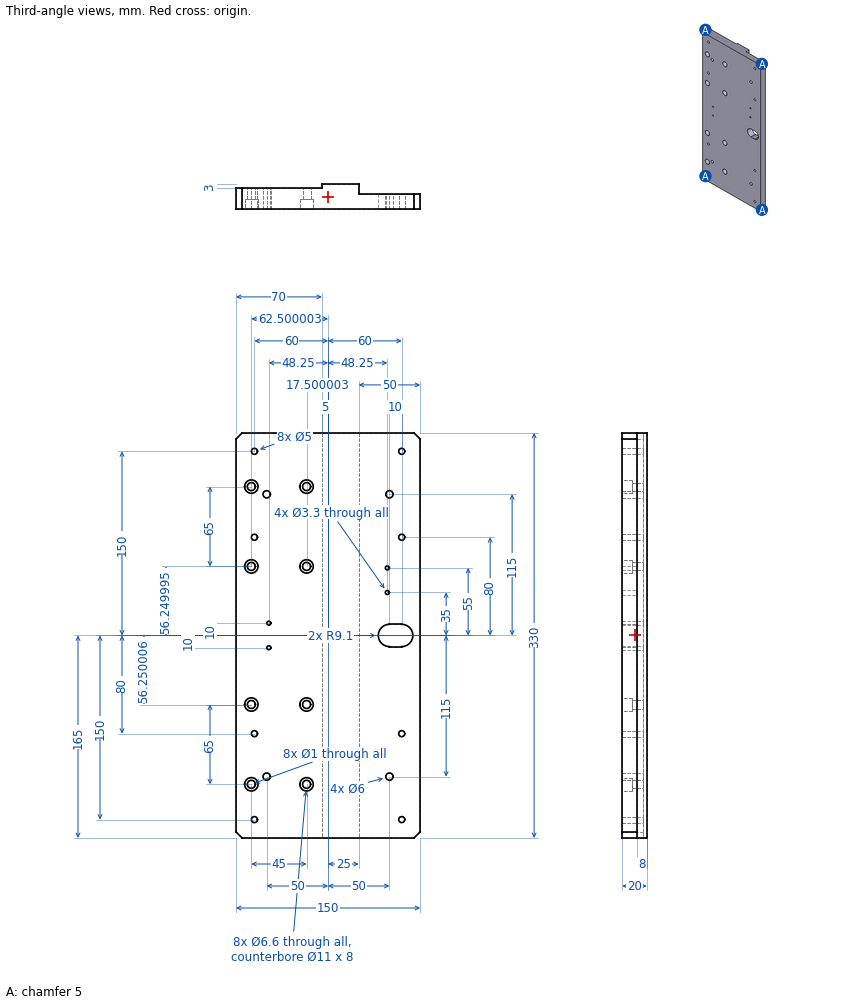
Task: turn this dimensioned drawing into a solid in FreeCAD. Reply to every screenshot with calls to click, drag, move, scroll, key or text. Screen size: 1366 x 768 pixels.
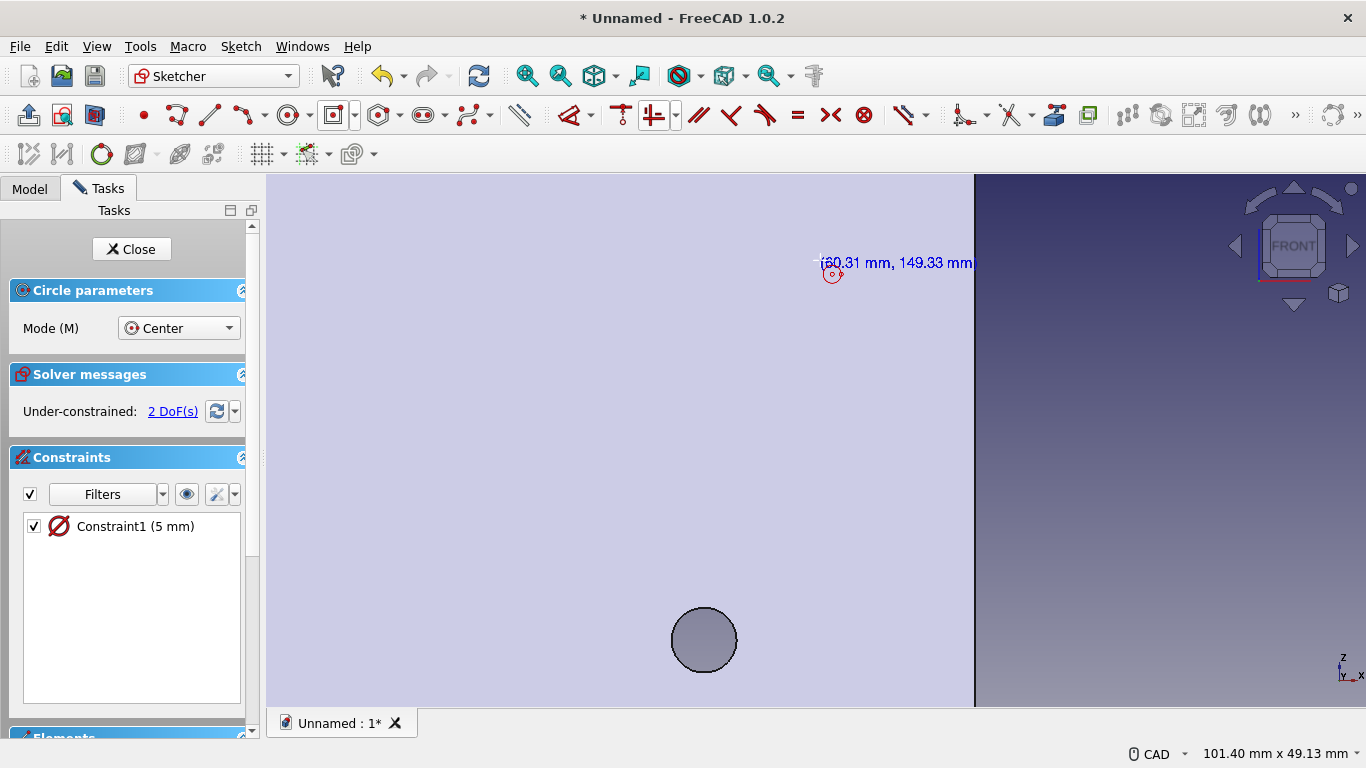
scroll(820, 260, down, 11)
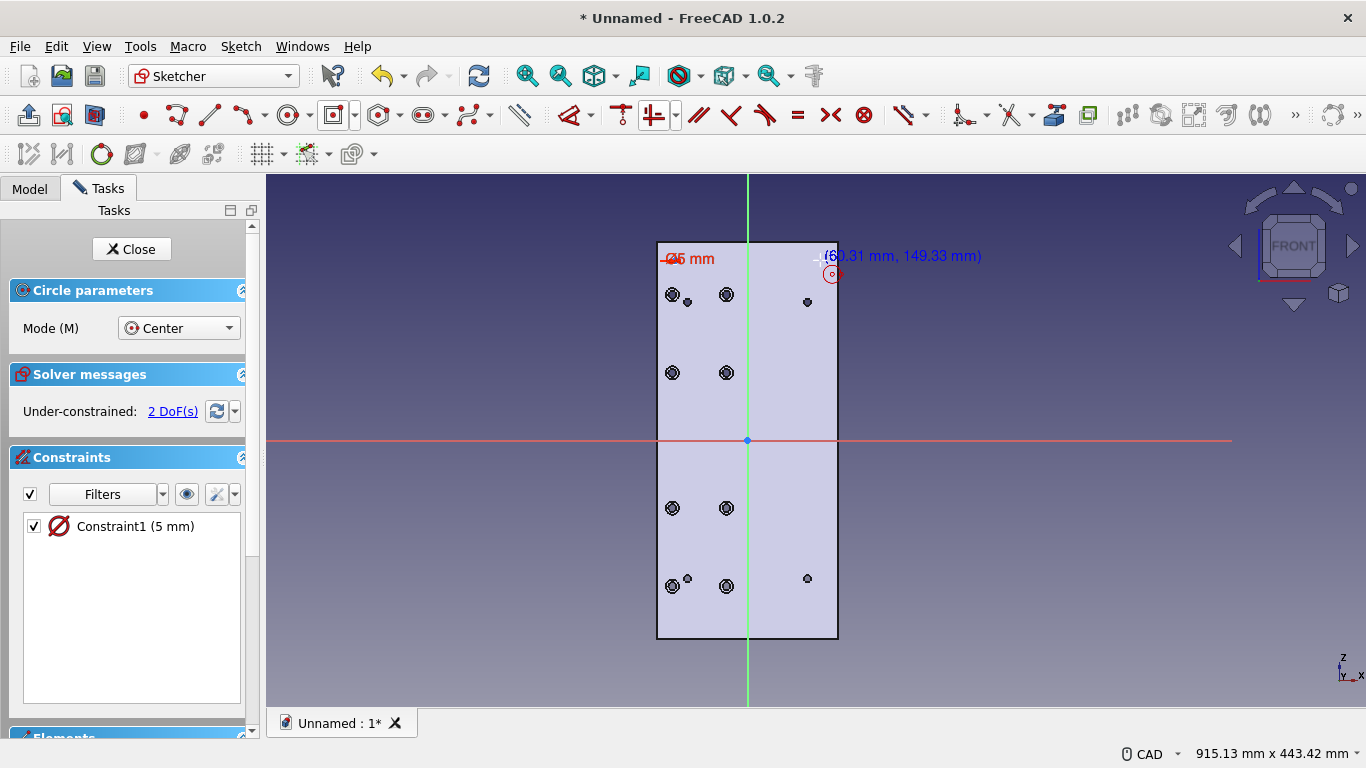
click(820, 260)
move(822, 258)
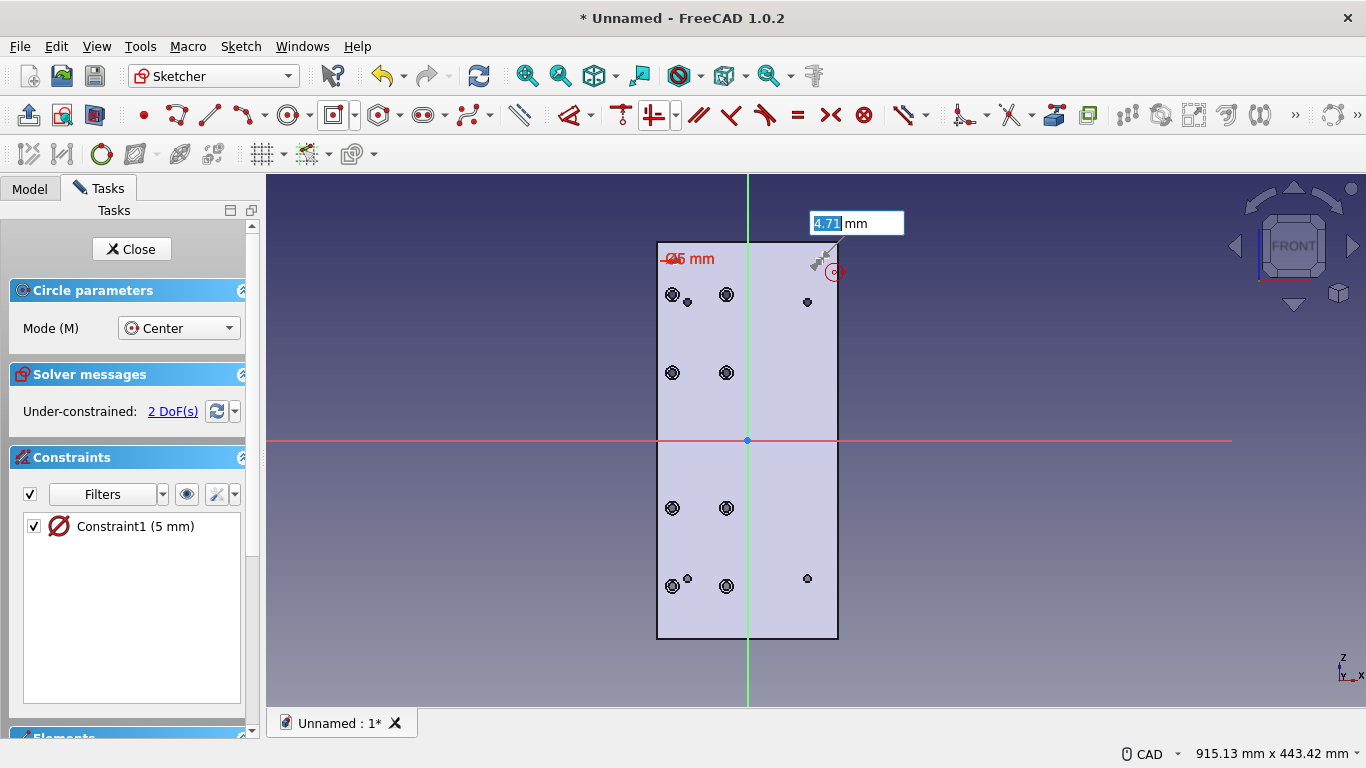
text(5)
key(Return)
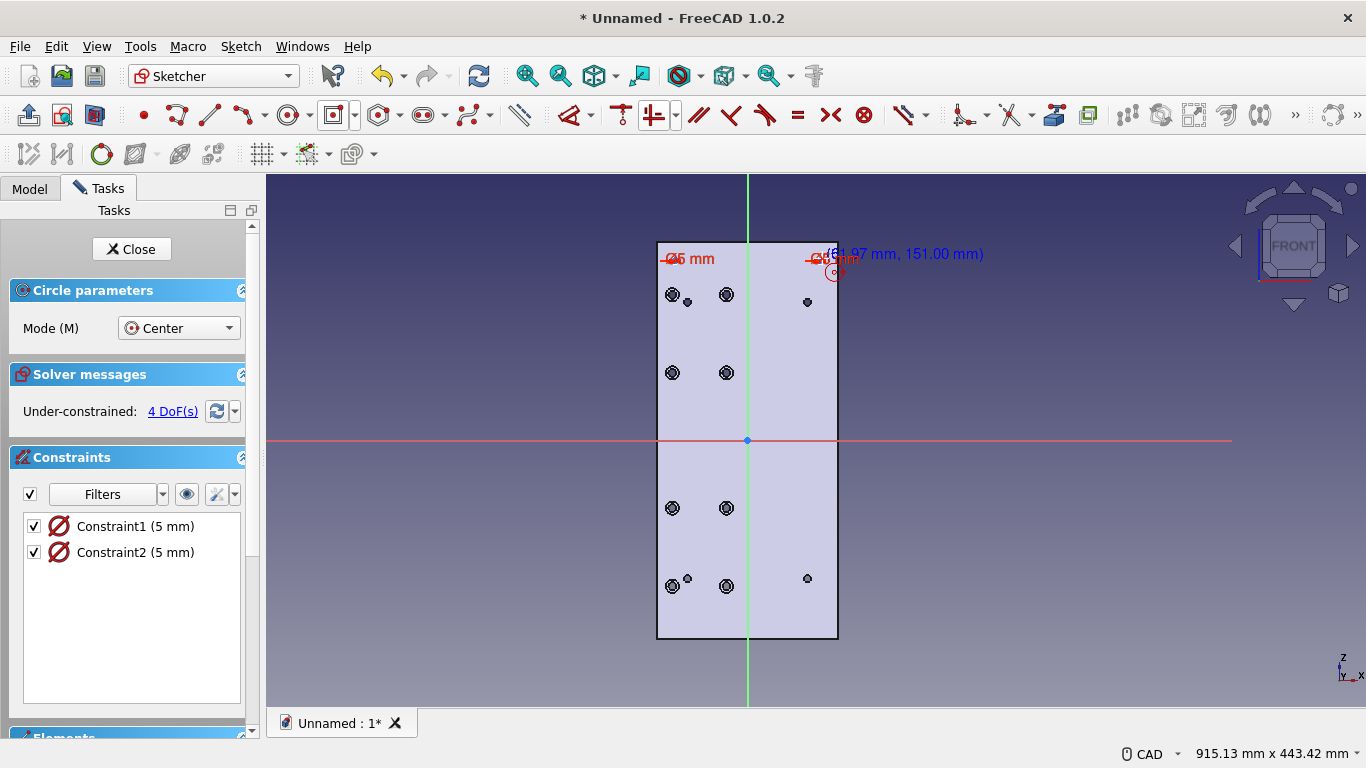
scroll(820, 344, up, 11)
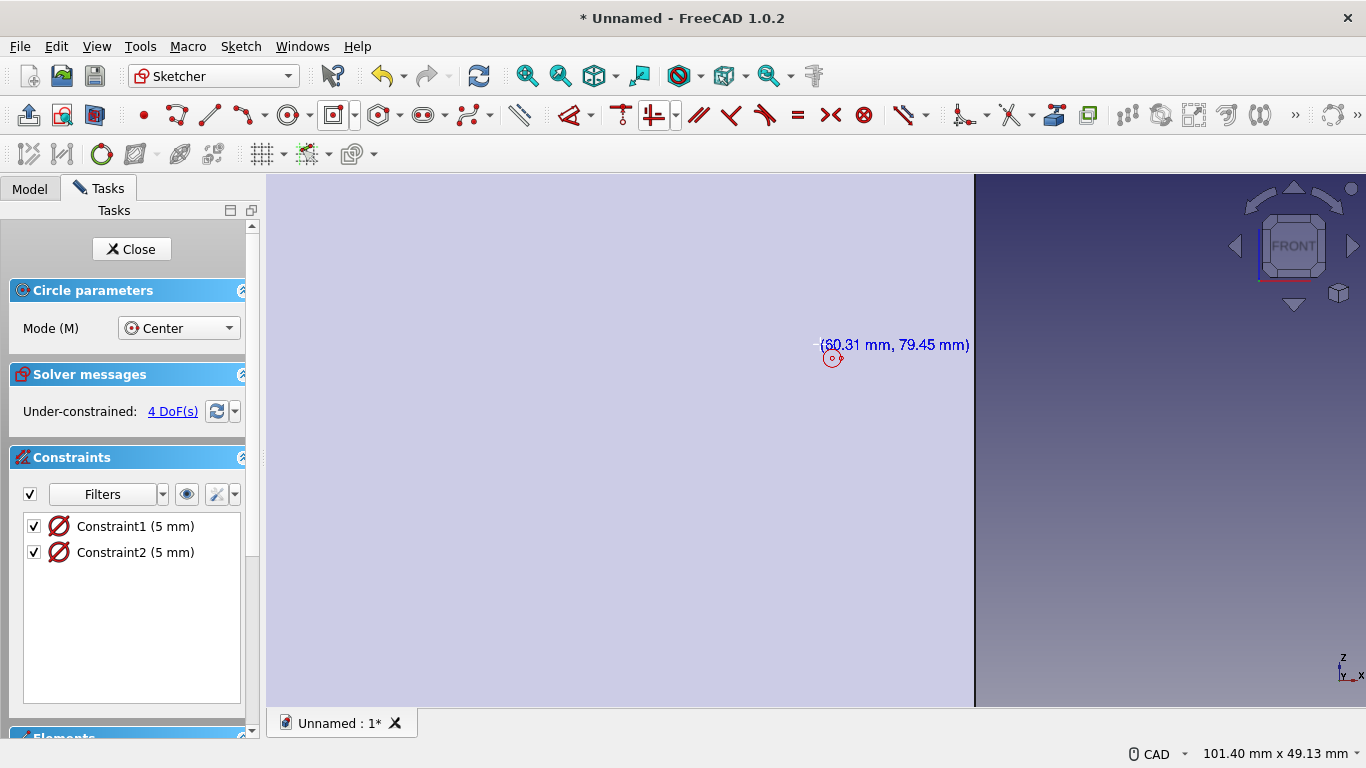
scroll(820, 344, down, 11)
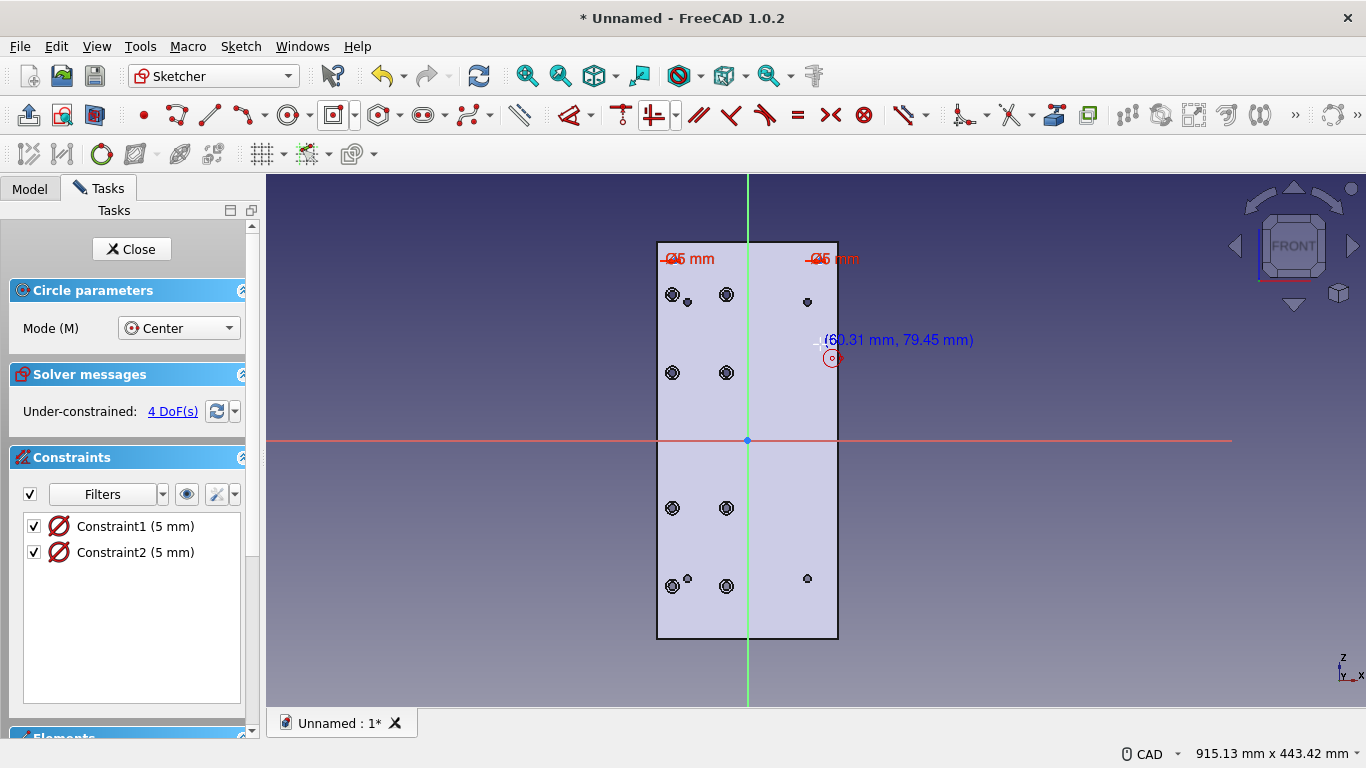
click(820, 344)
move(822, 342)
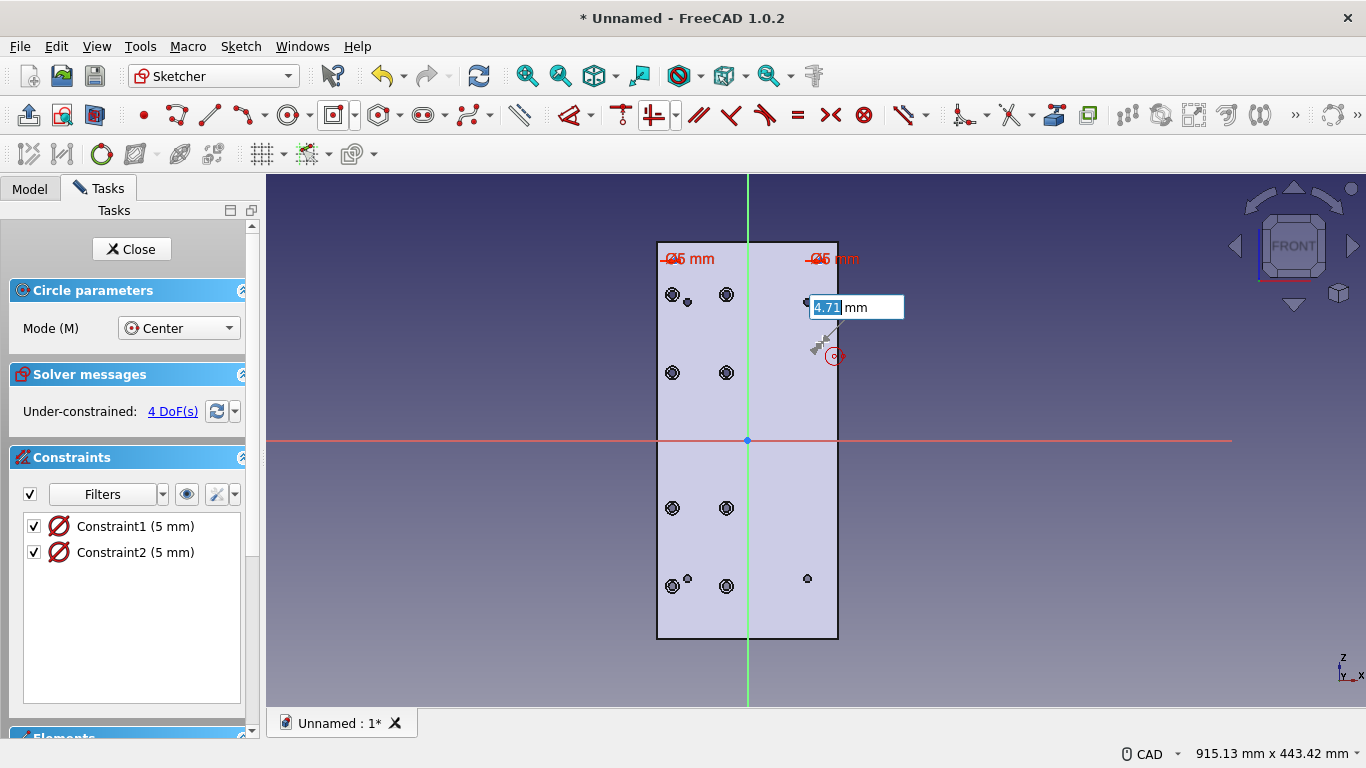
text(5)
key(Return)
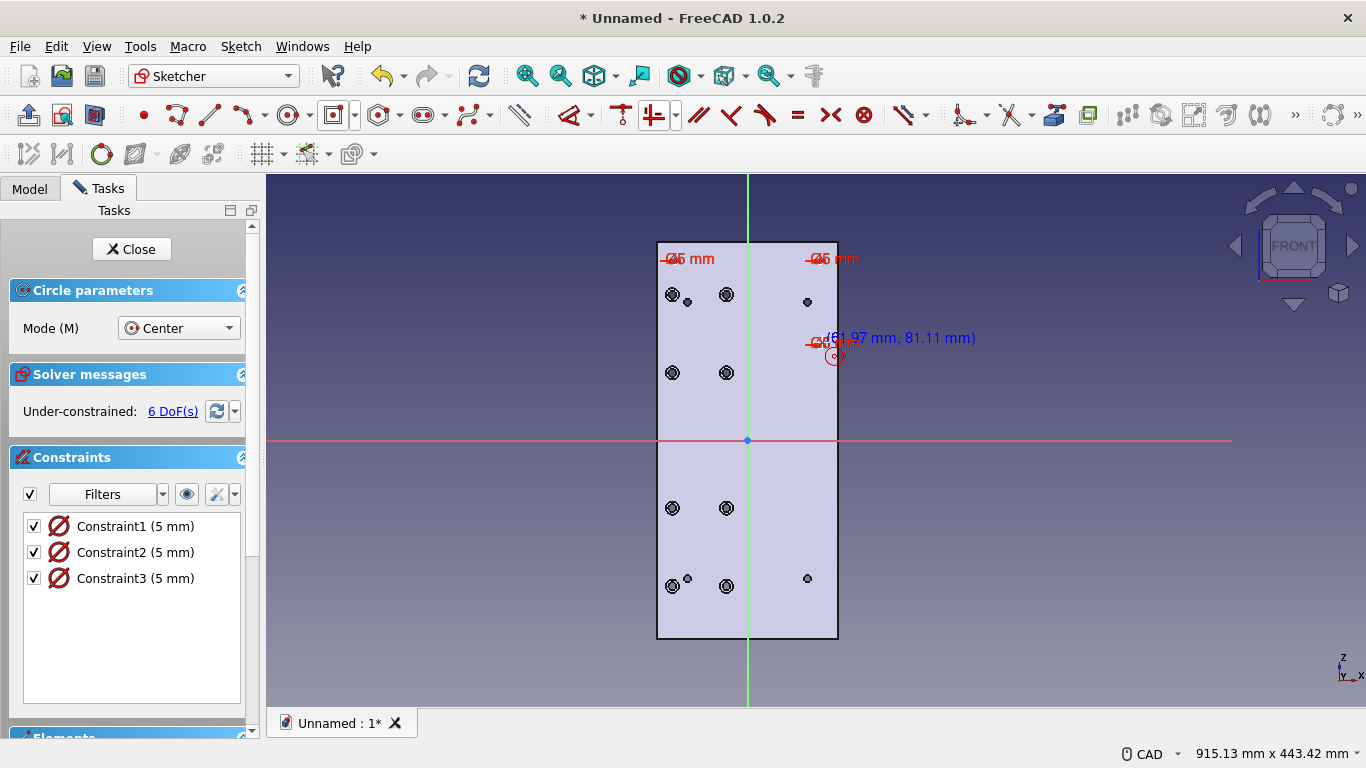
scroll(675, 344, up, 11)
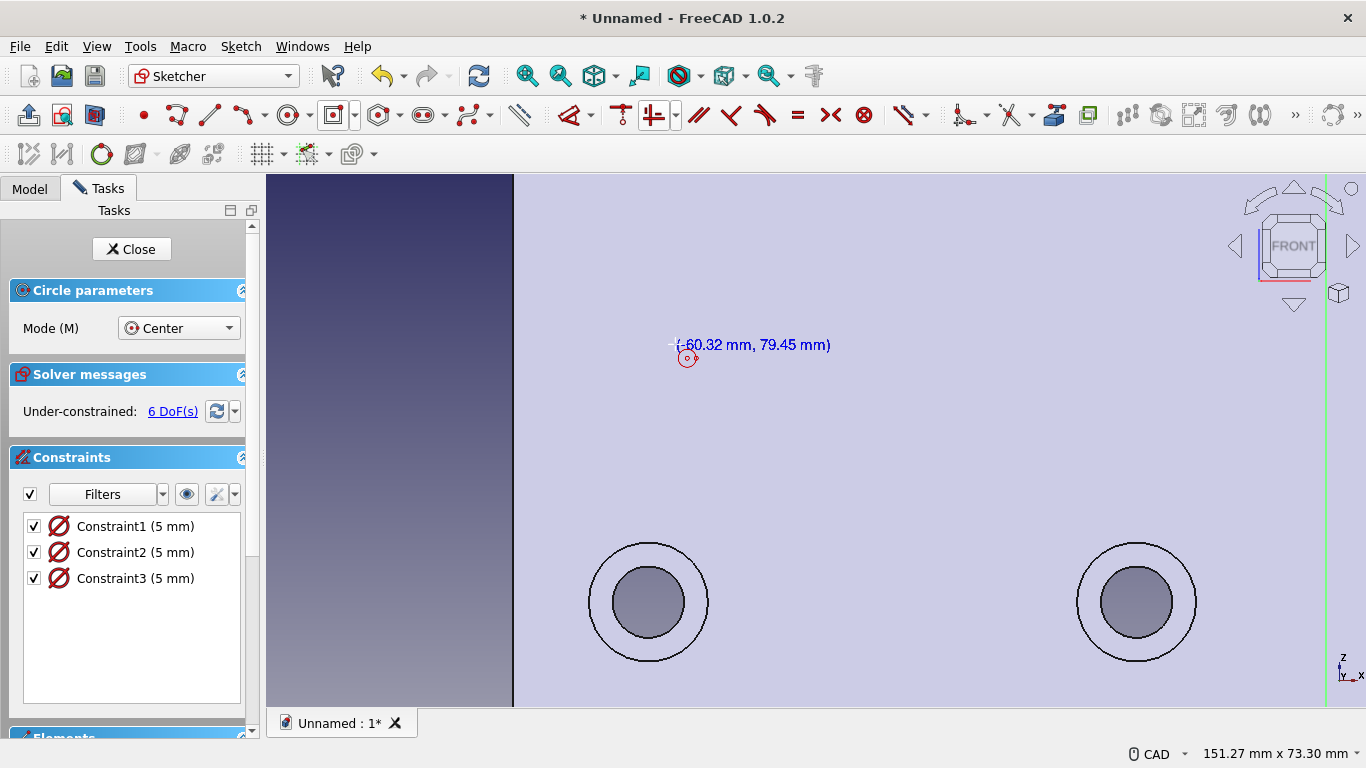
scroll(675, 344, down, 11)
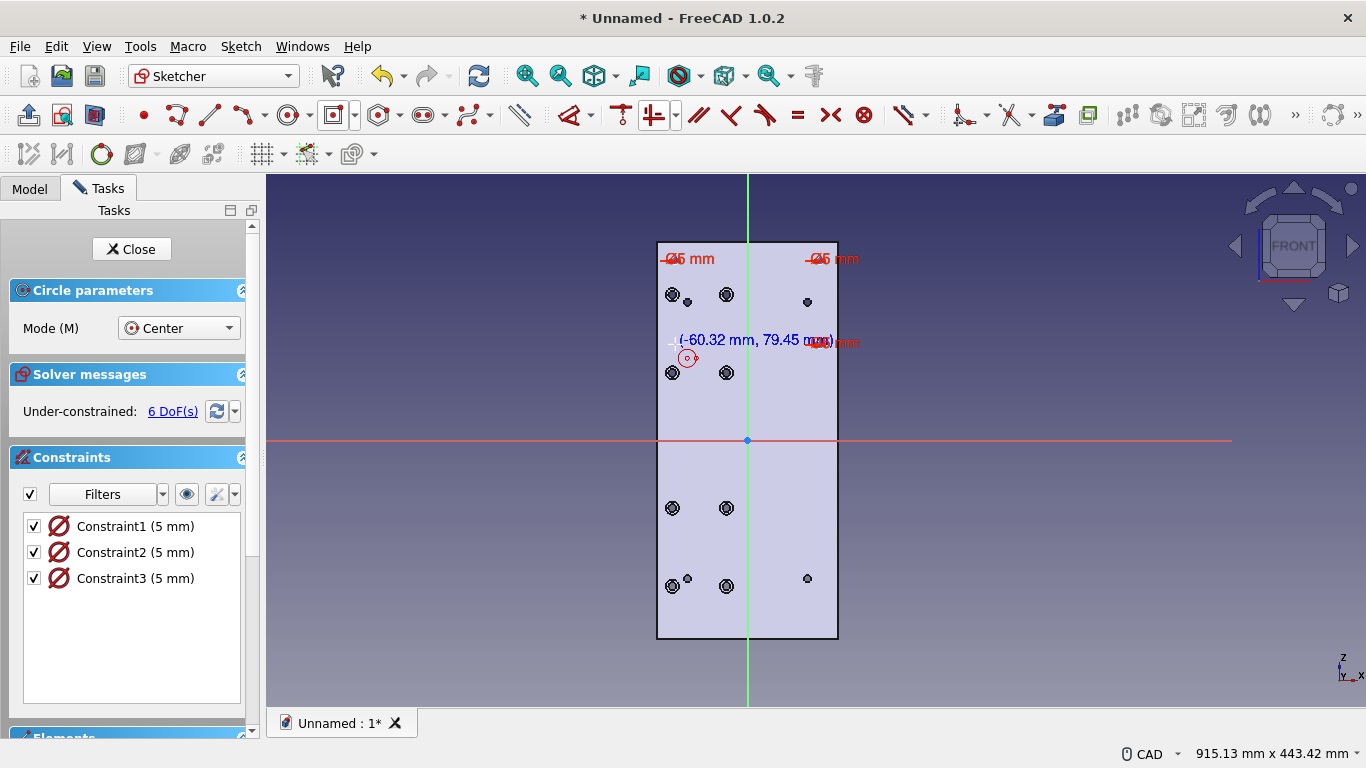
click(675, 344)
move(678, 342)